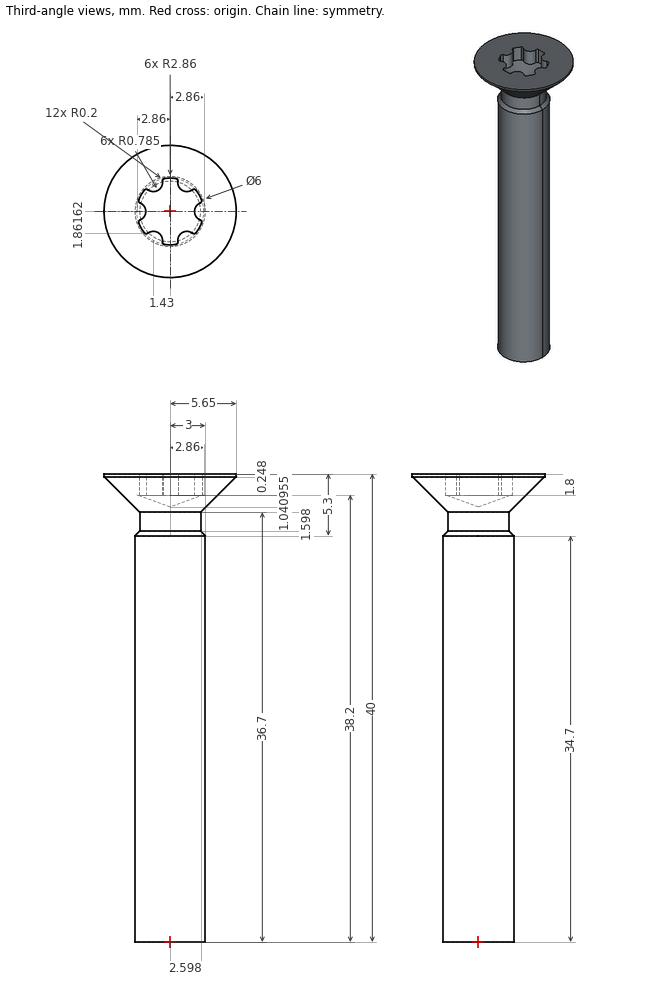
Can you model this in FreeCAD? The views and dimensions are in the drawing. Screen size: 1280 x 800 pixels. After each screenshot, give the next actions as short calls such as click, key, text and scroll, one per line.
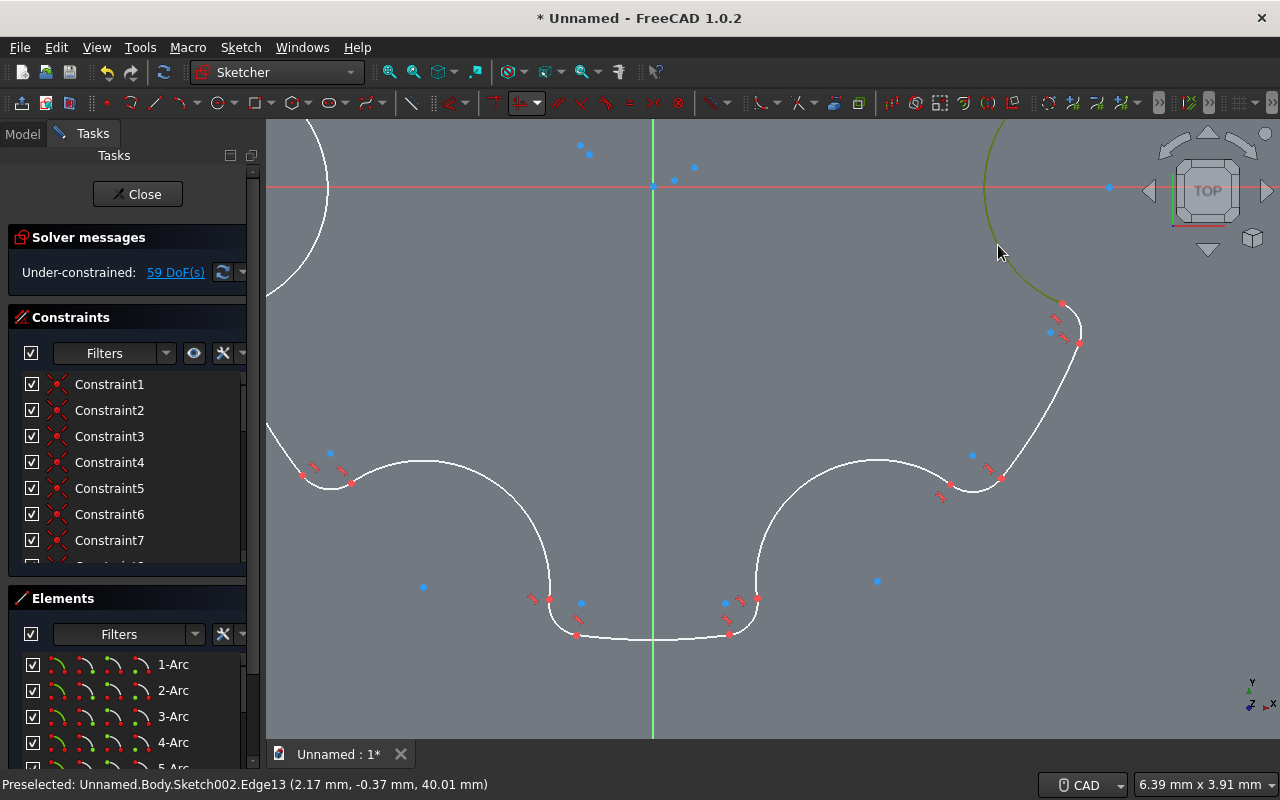
scroll(746, 627, down, 4)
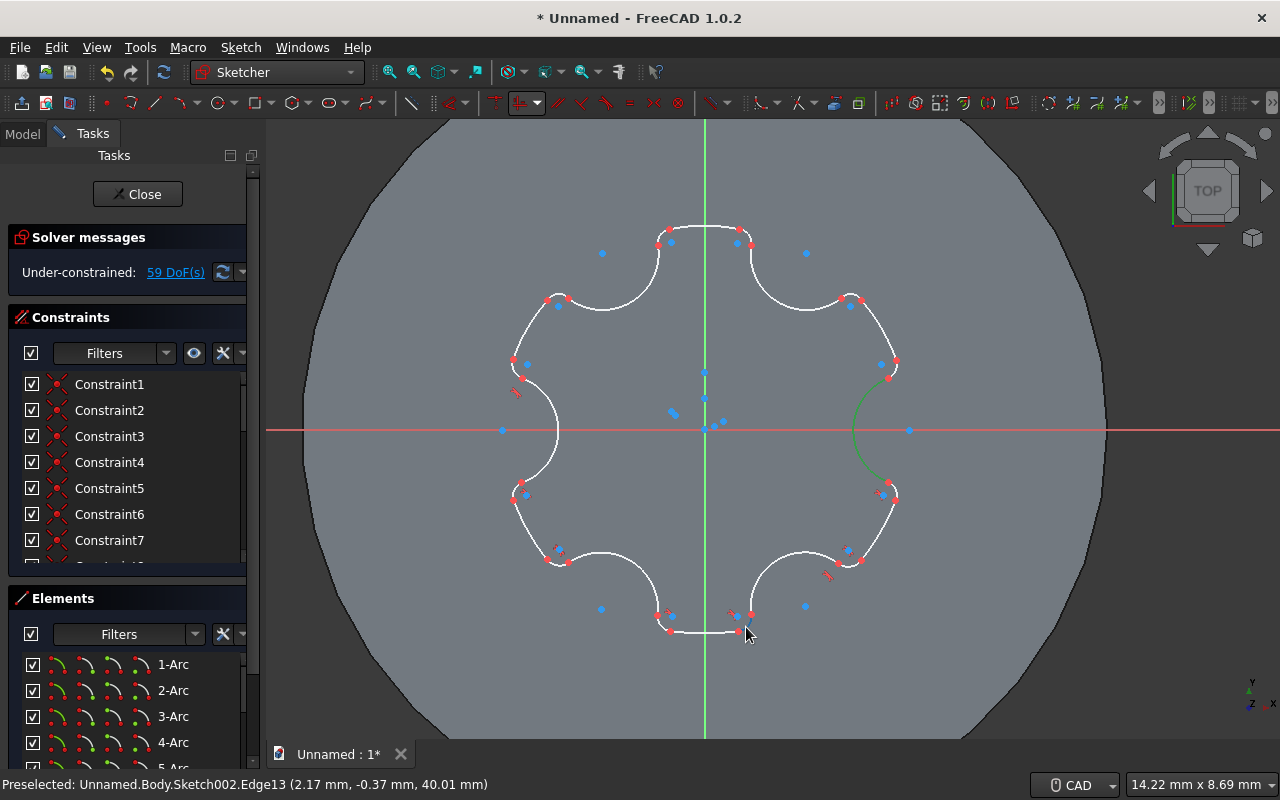
scroll(893, 374, up, 4)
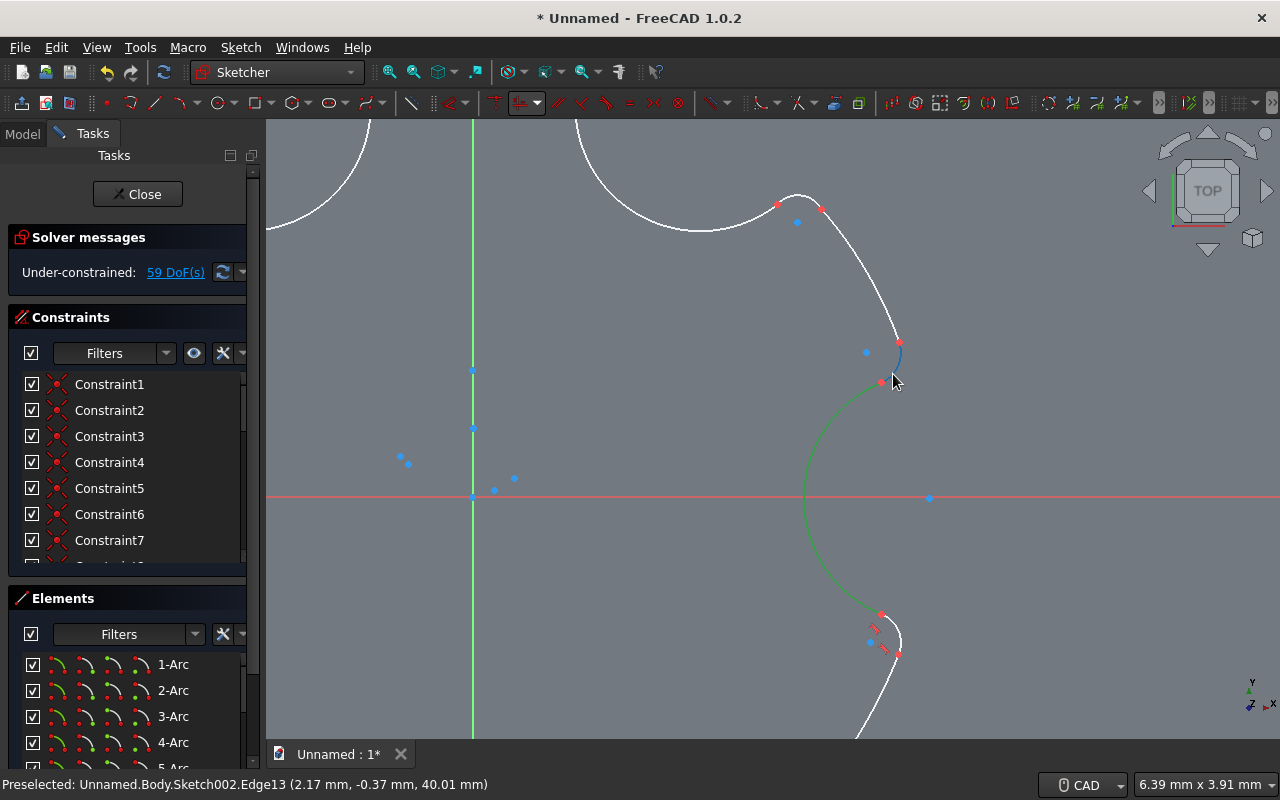
click(893, 374)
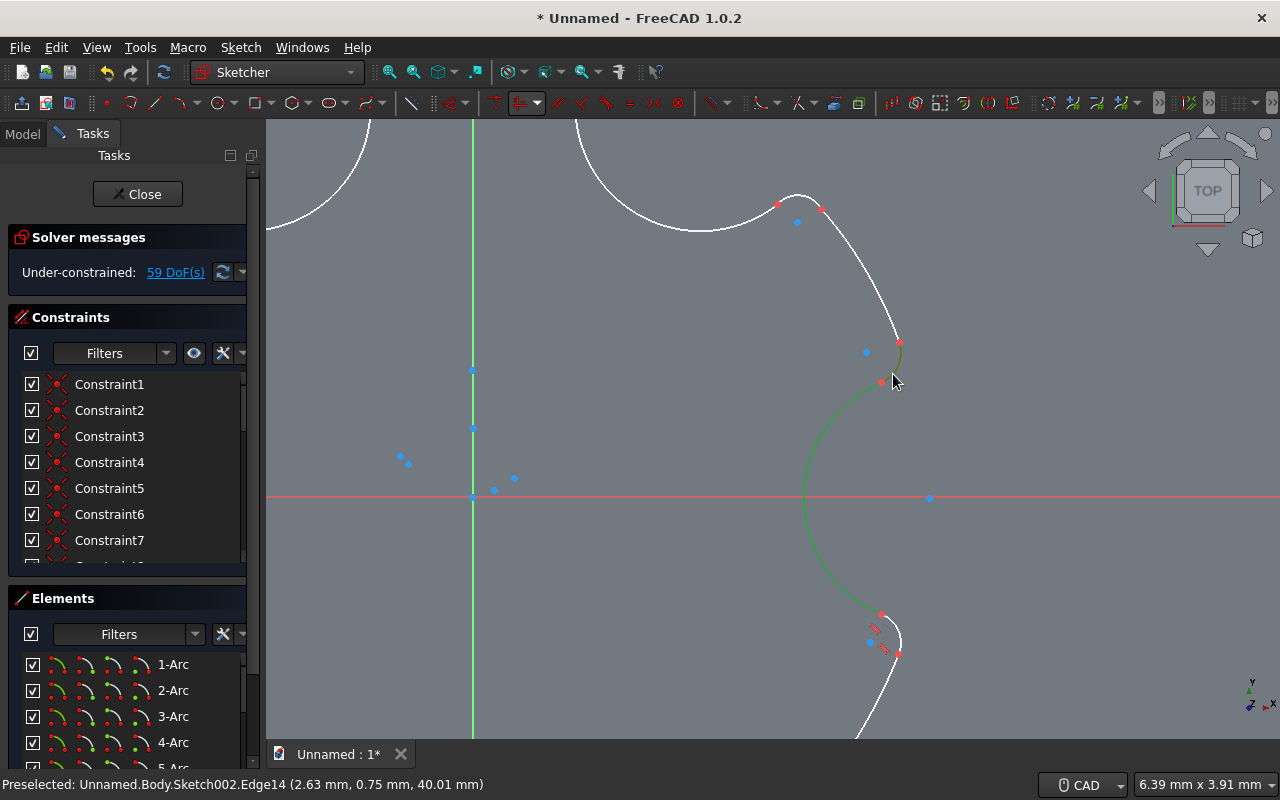
click(606, 104)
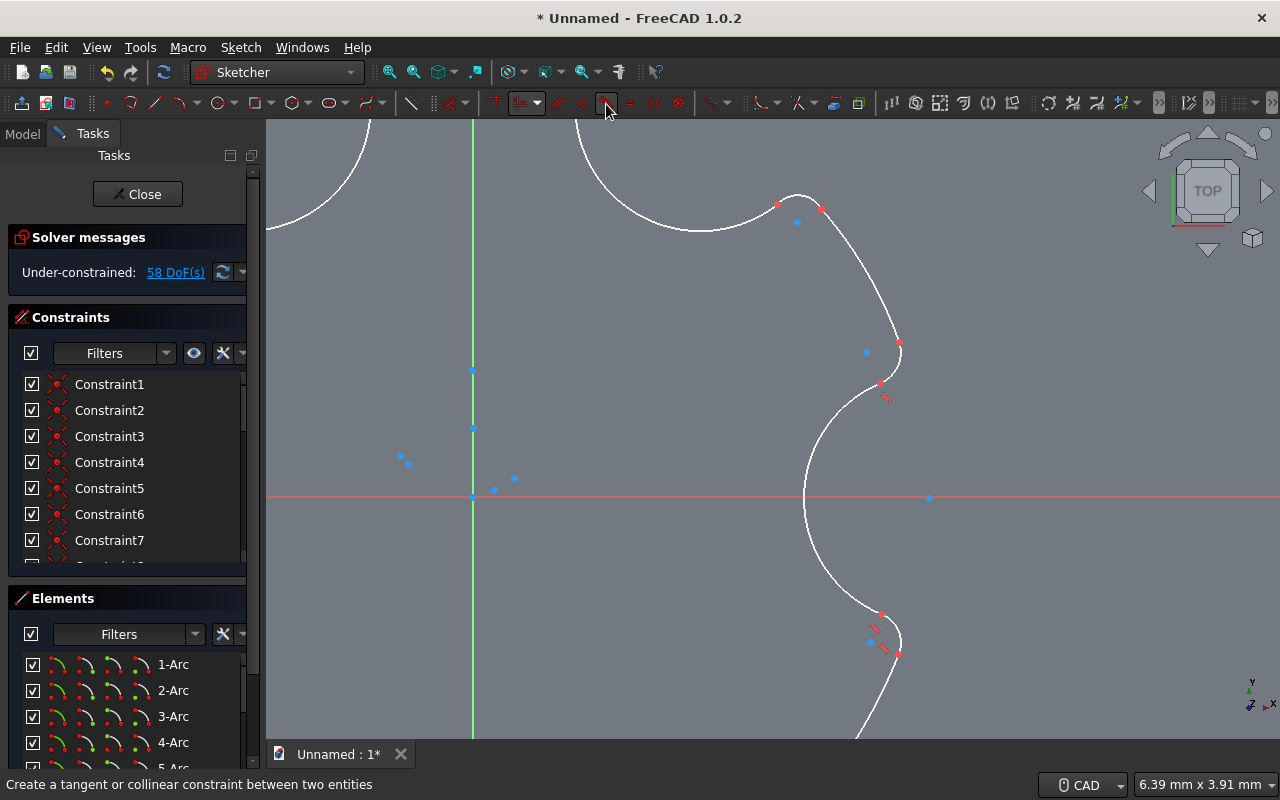
click(892, 375)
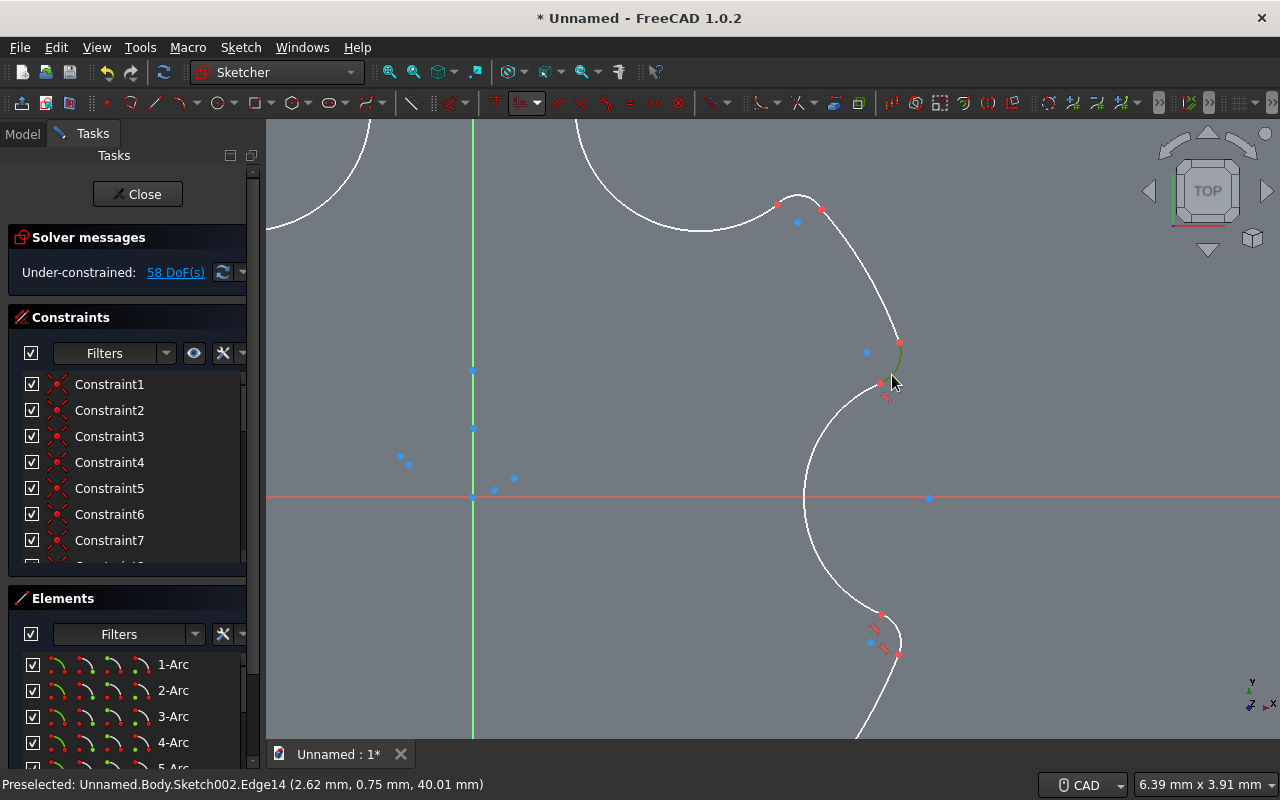
click(882, 300)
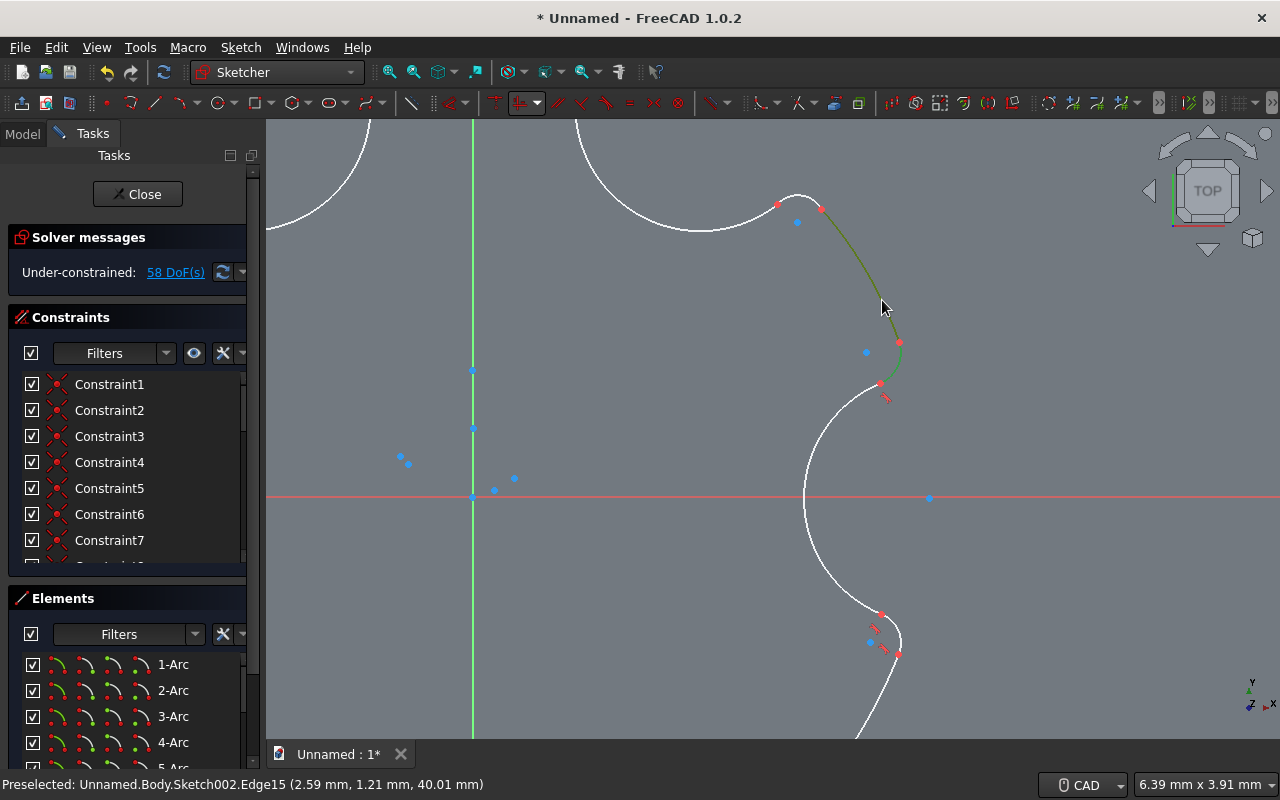
click(606, 104)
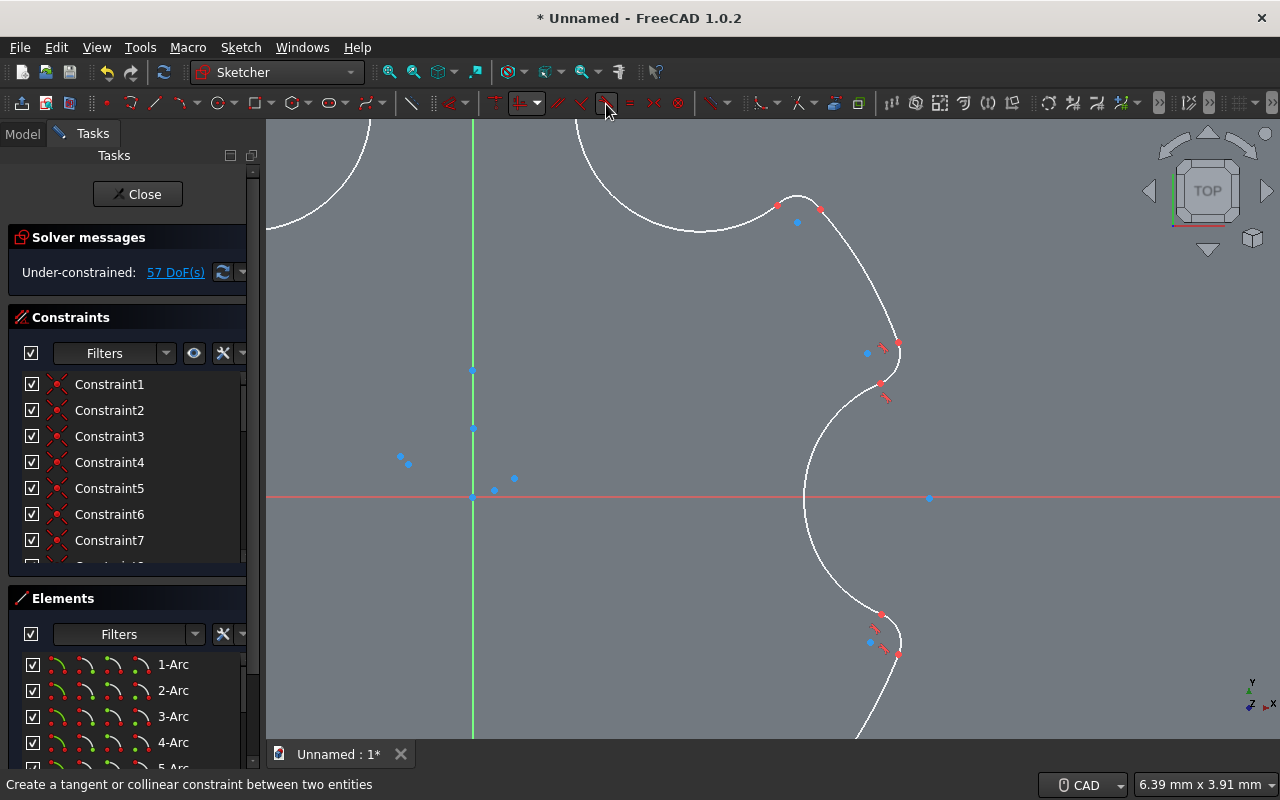
click(880, 300)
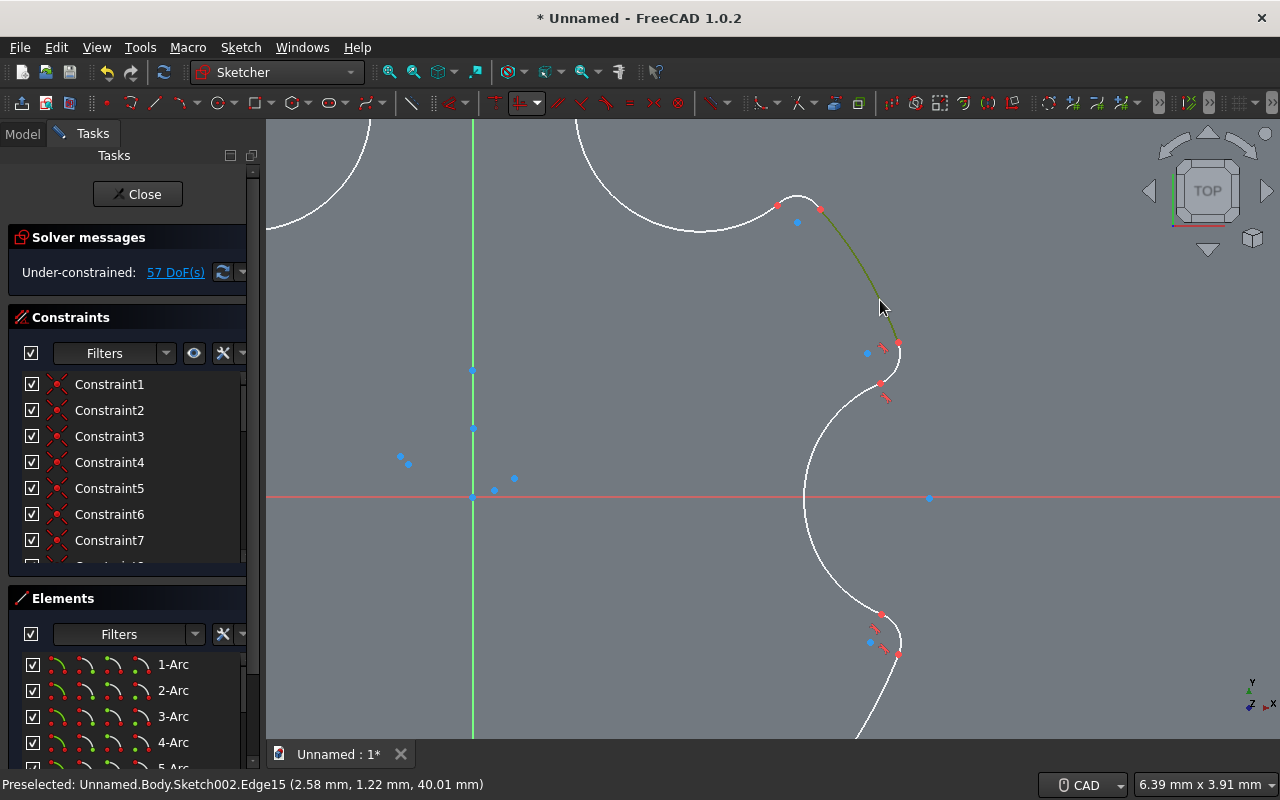
click(809, 199)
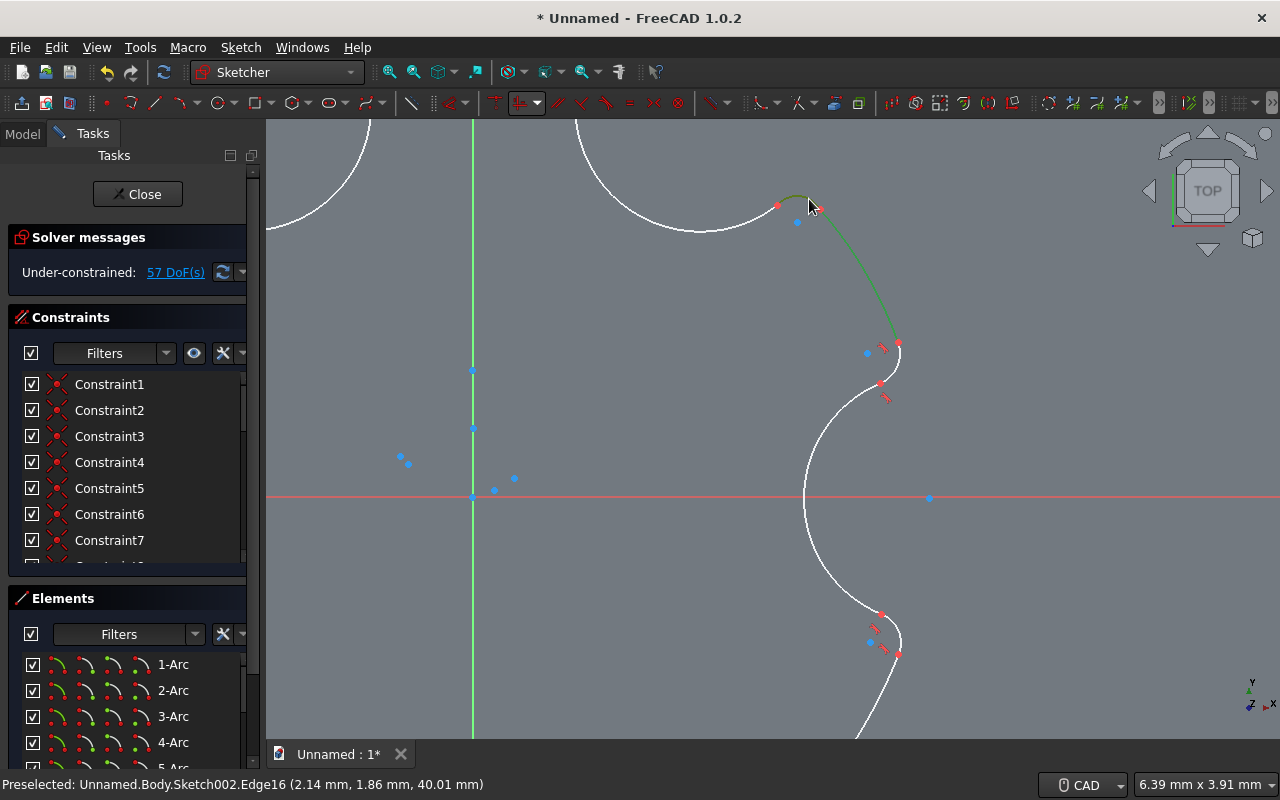
key(t)